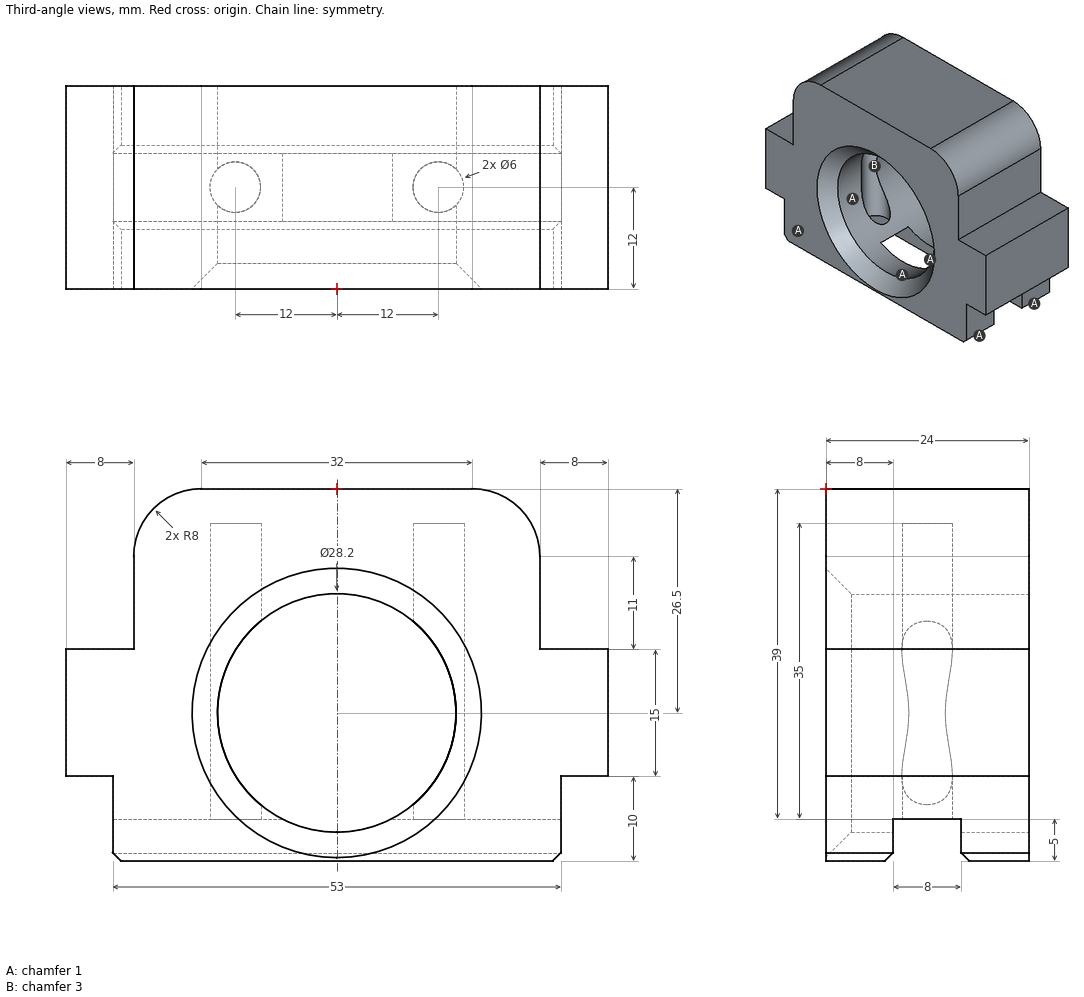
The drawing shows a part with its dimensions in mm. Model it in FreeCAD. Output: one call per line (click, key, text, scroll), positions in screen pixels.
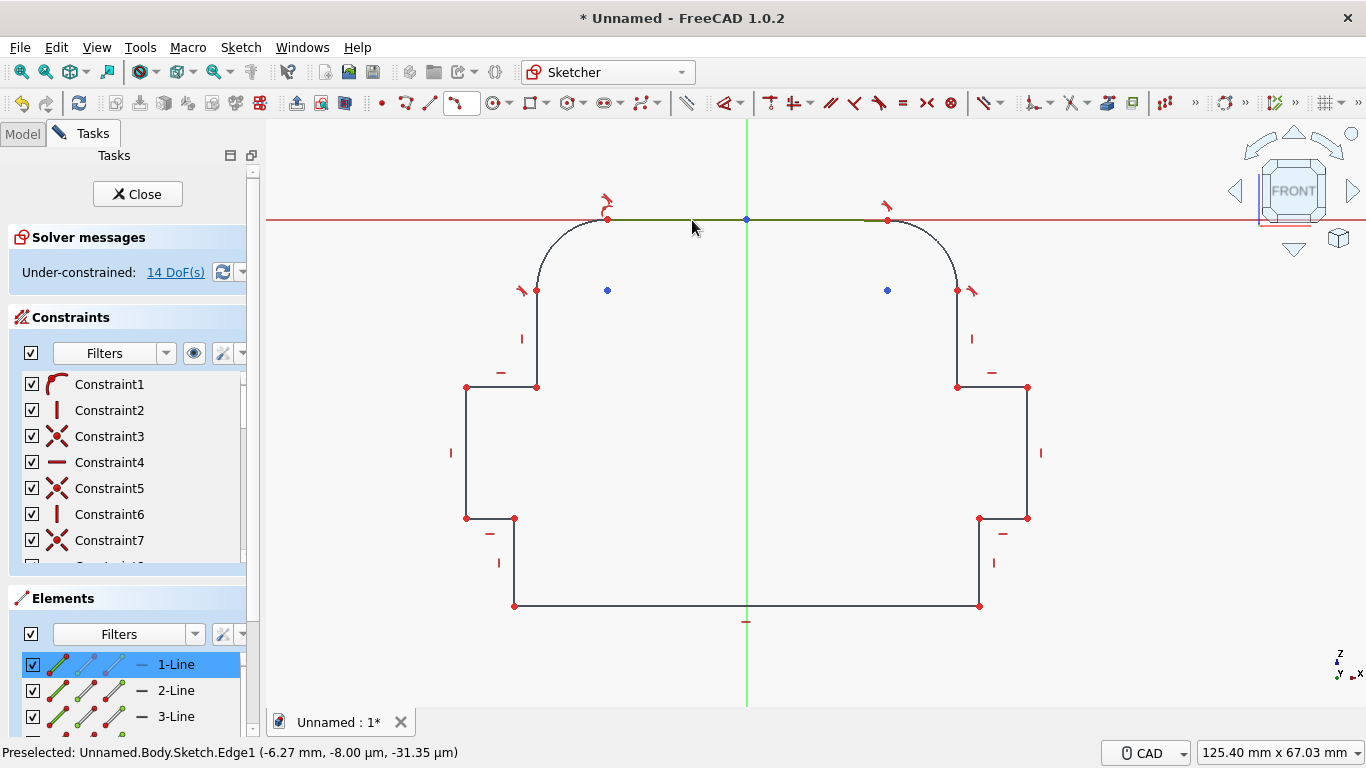
key(h)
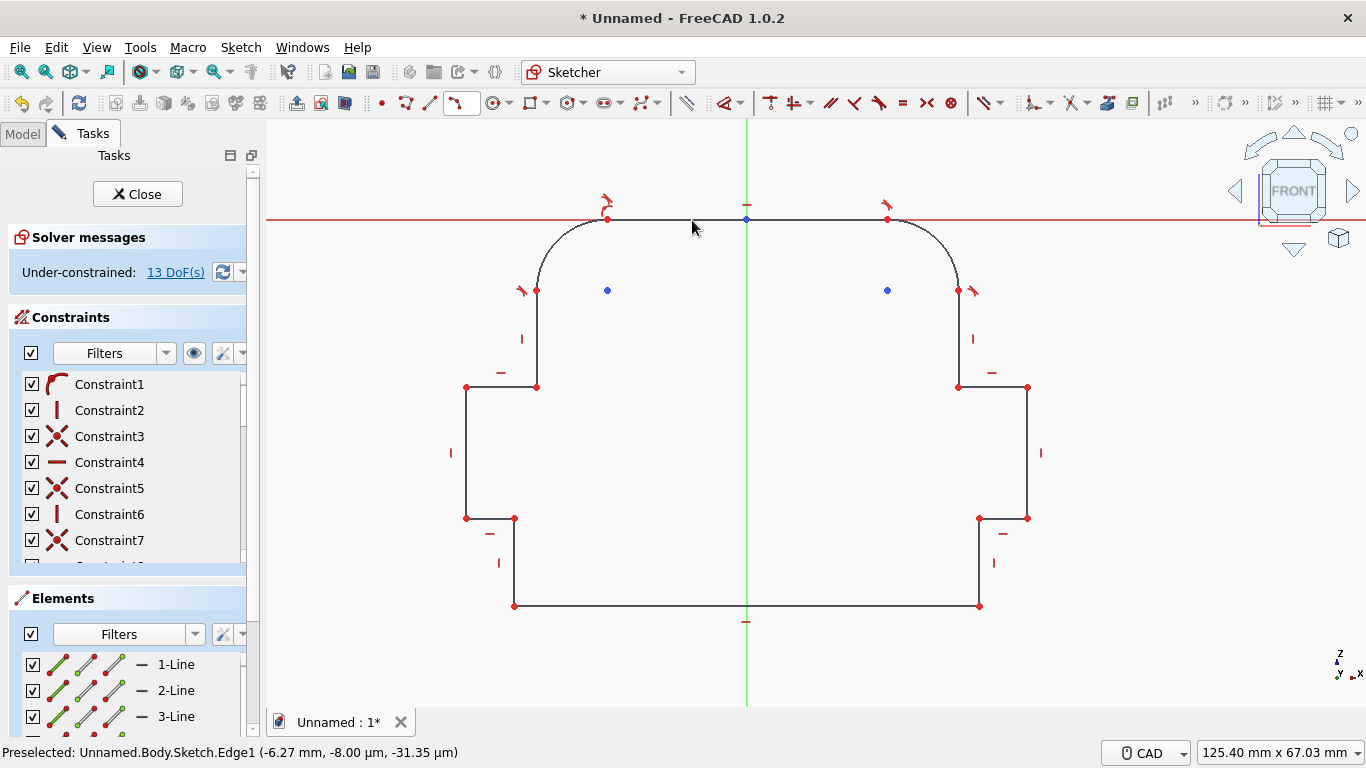
click(951, 258)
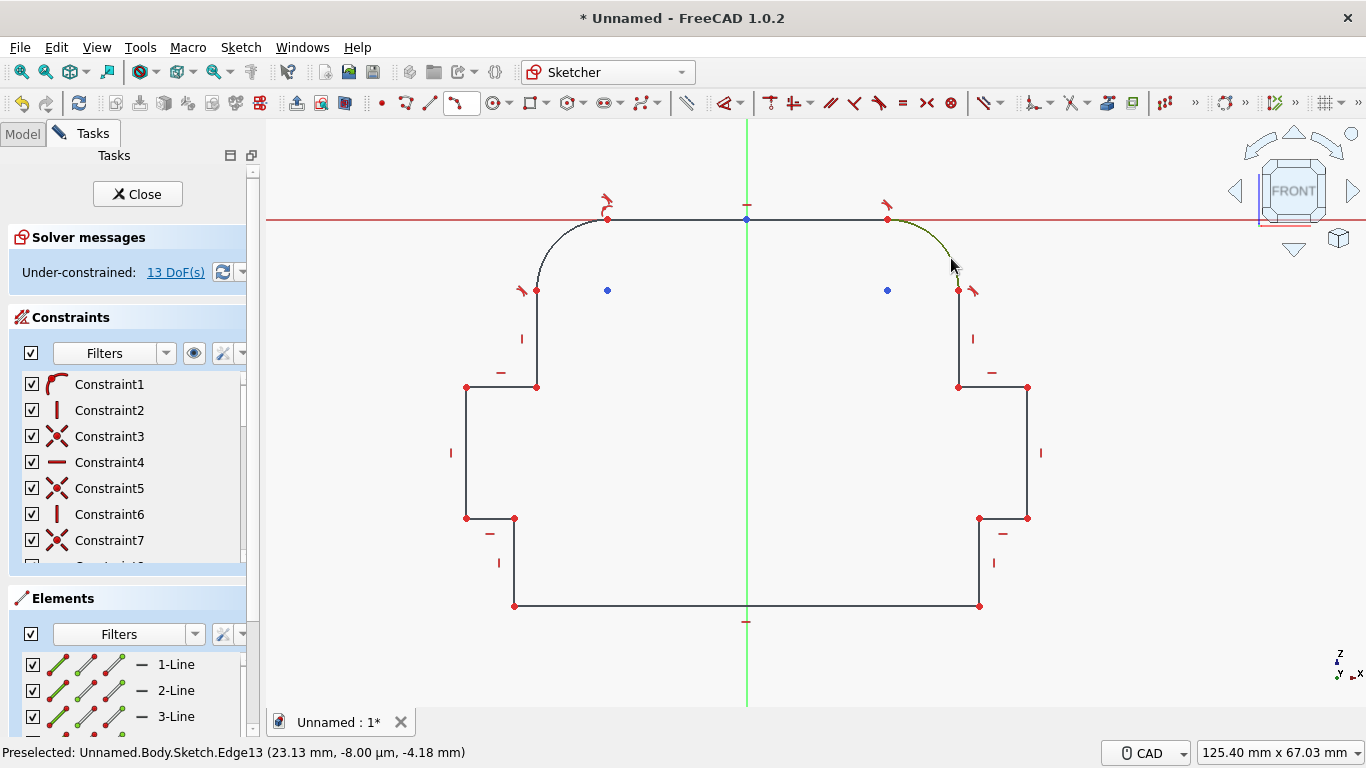
click(545, 258)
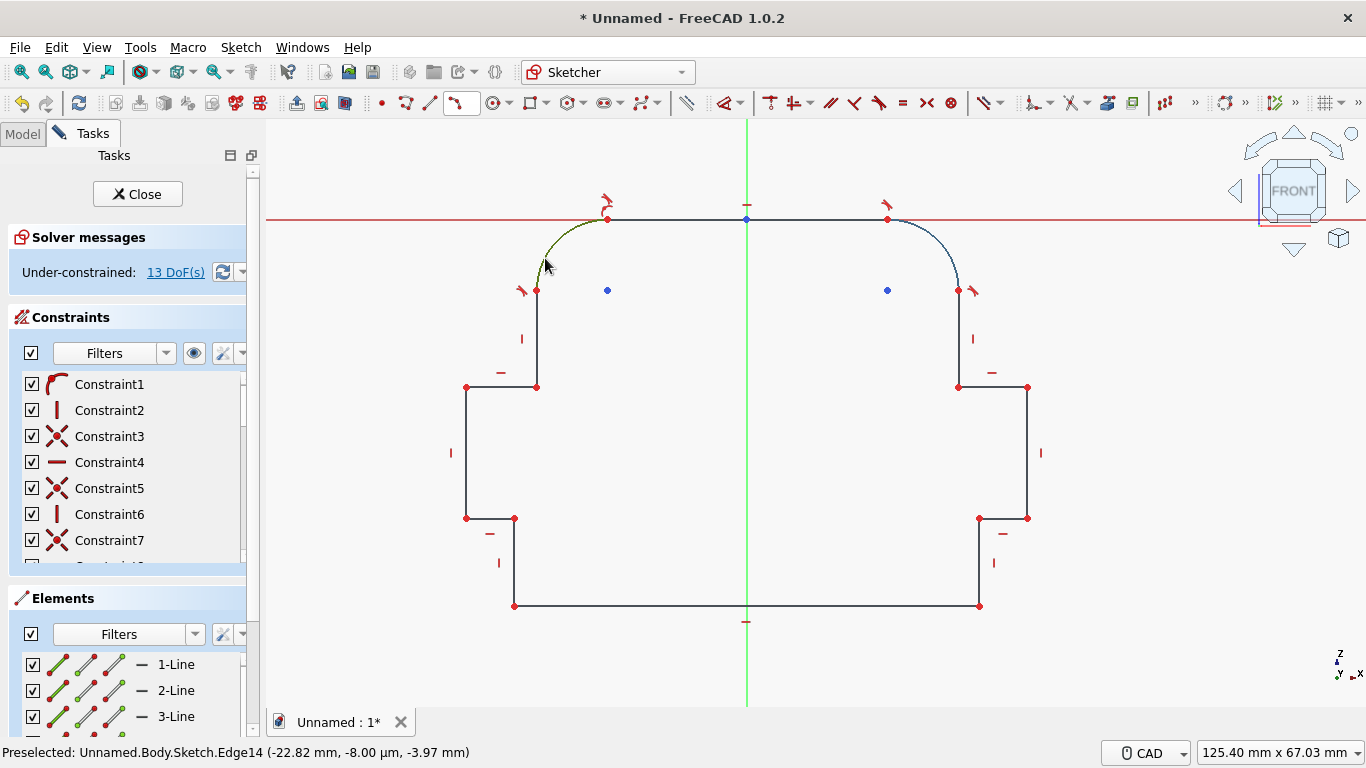
click(904, 104)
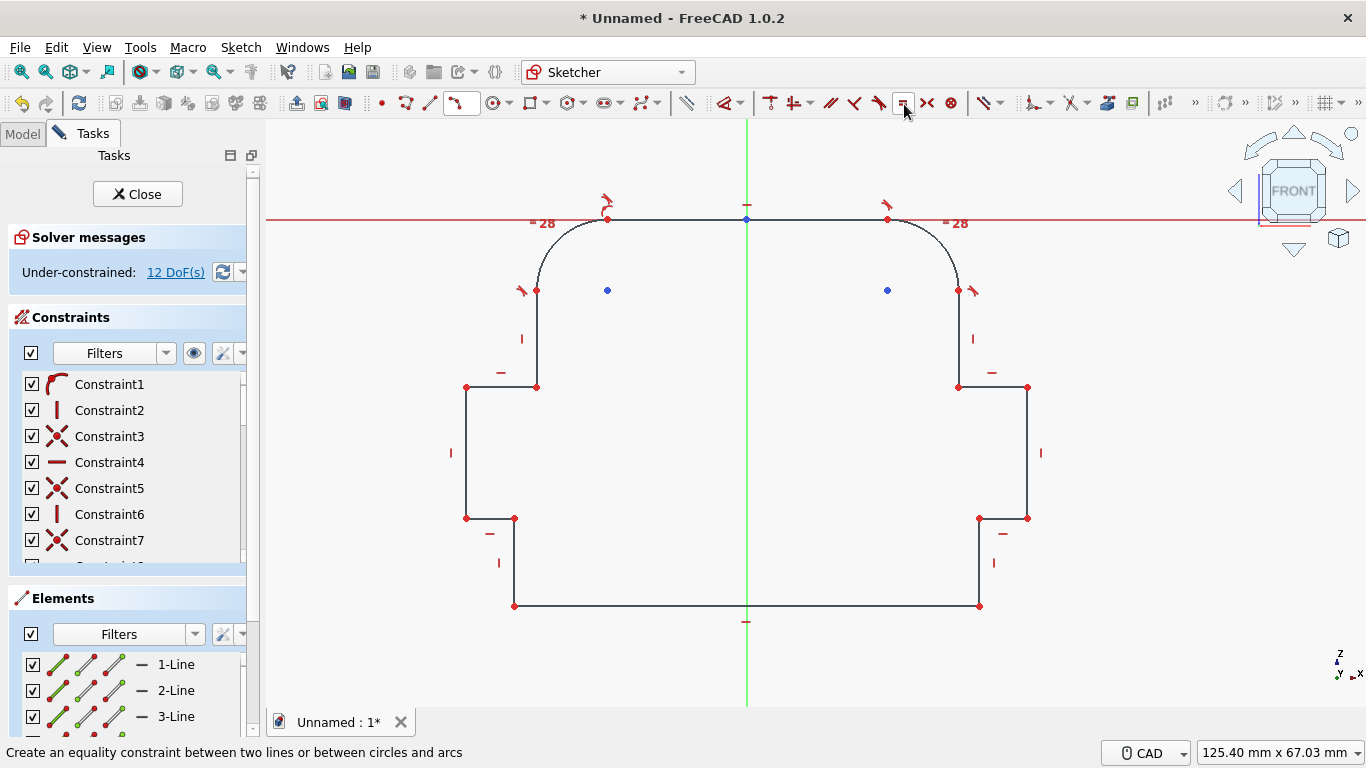
click(979, 519)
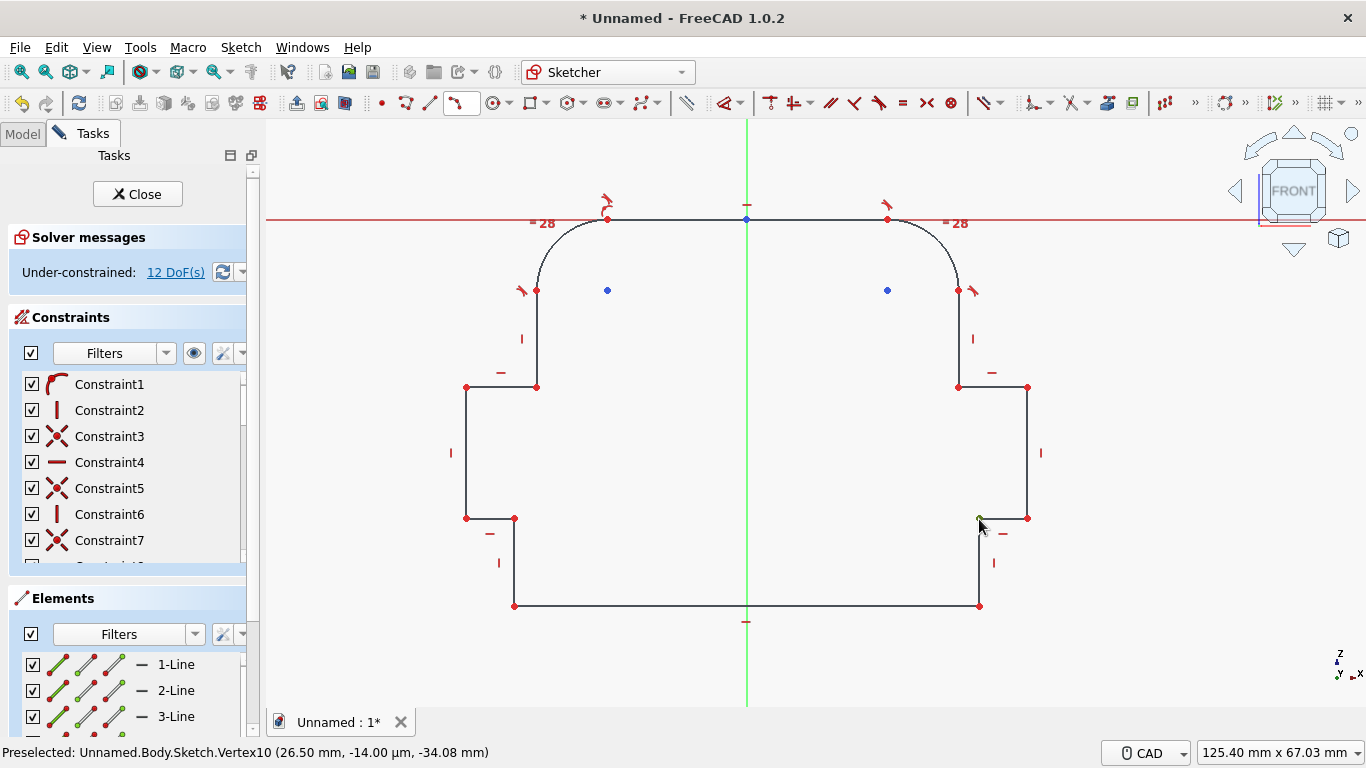
click(514, 519)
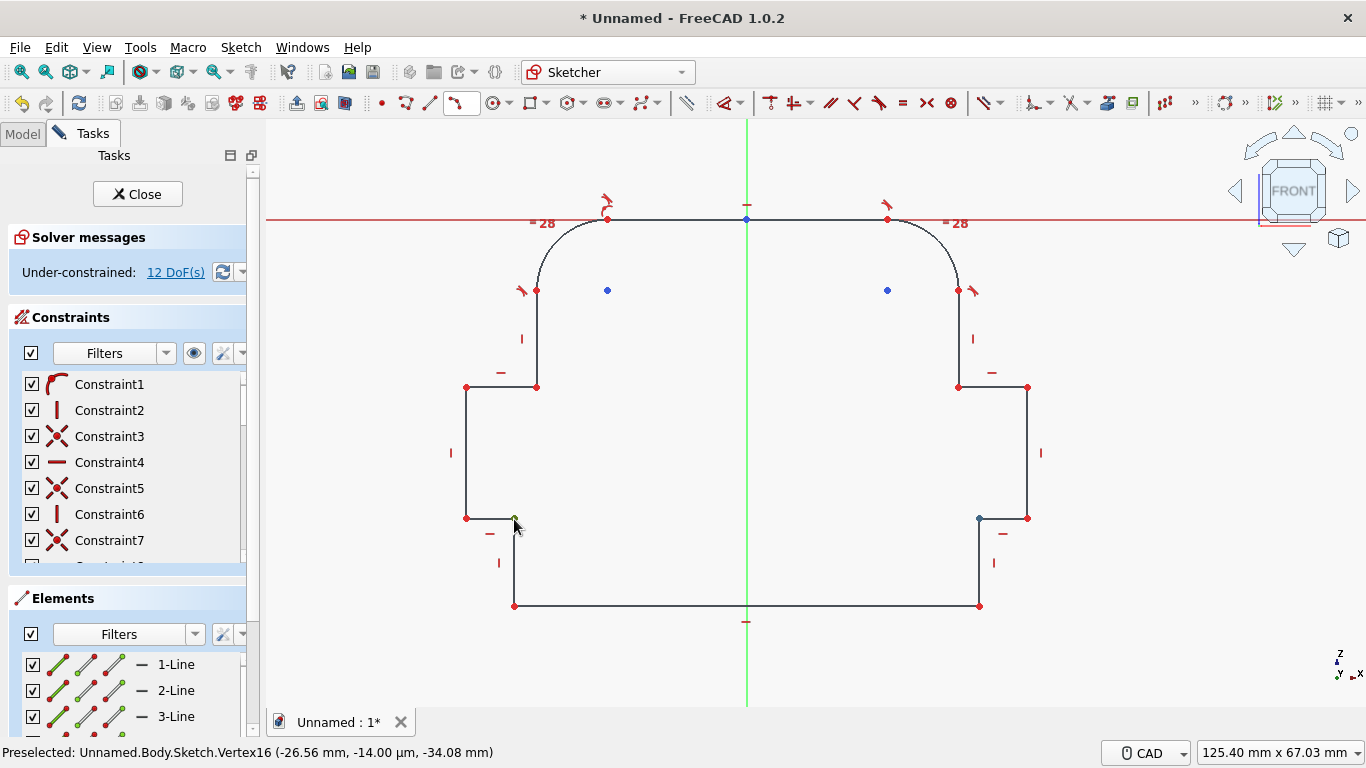
click(747, 641)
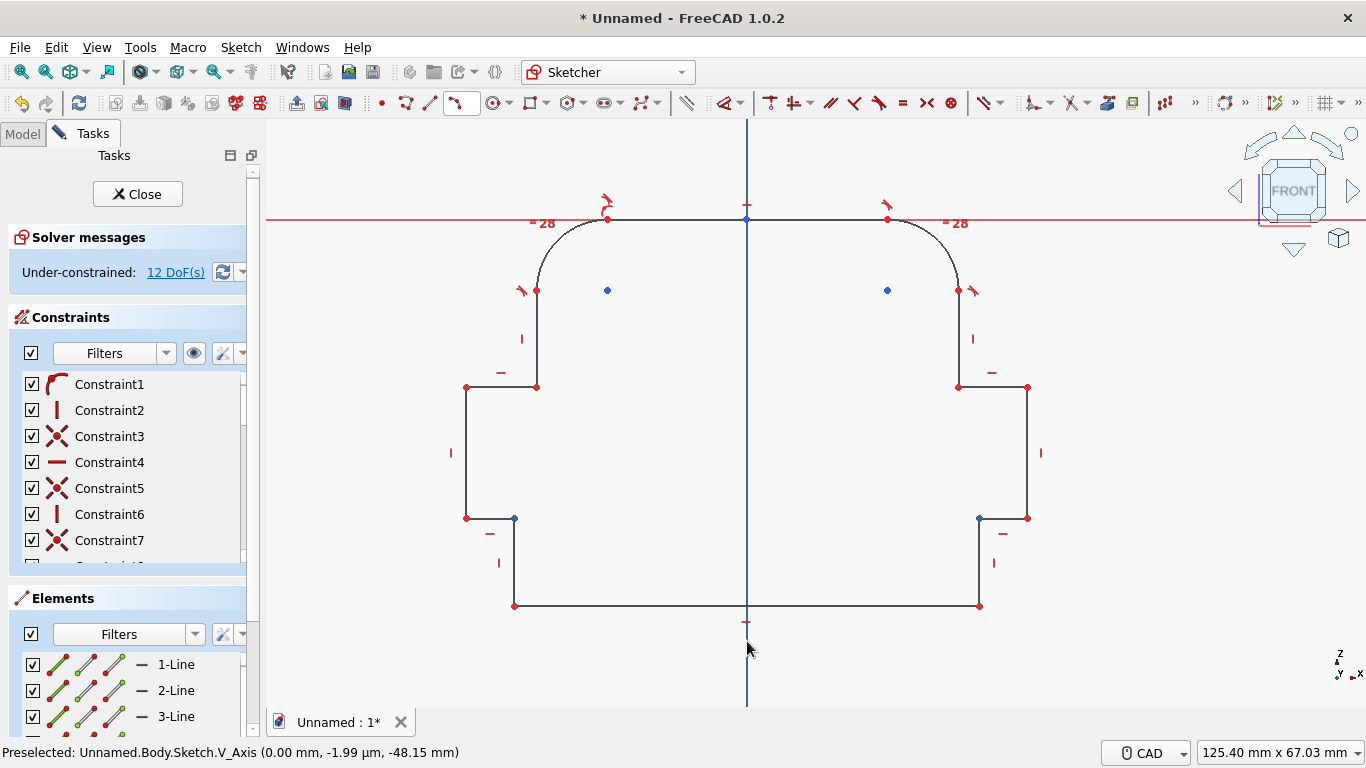
click(928, 104)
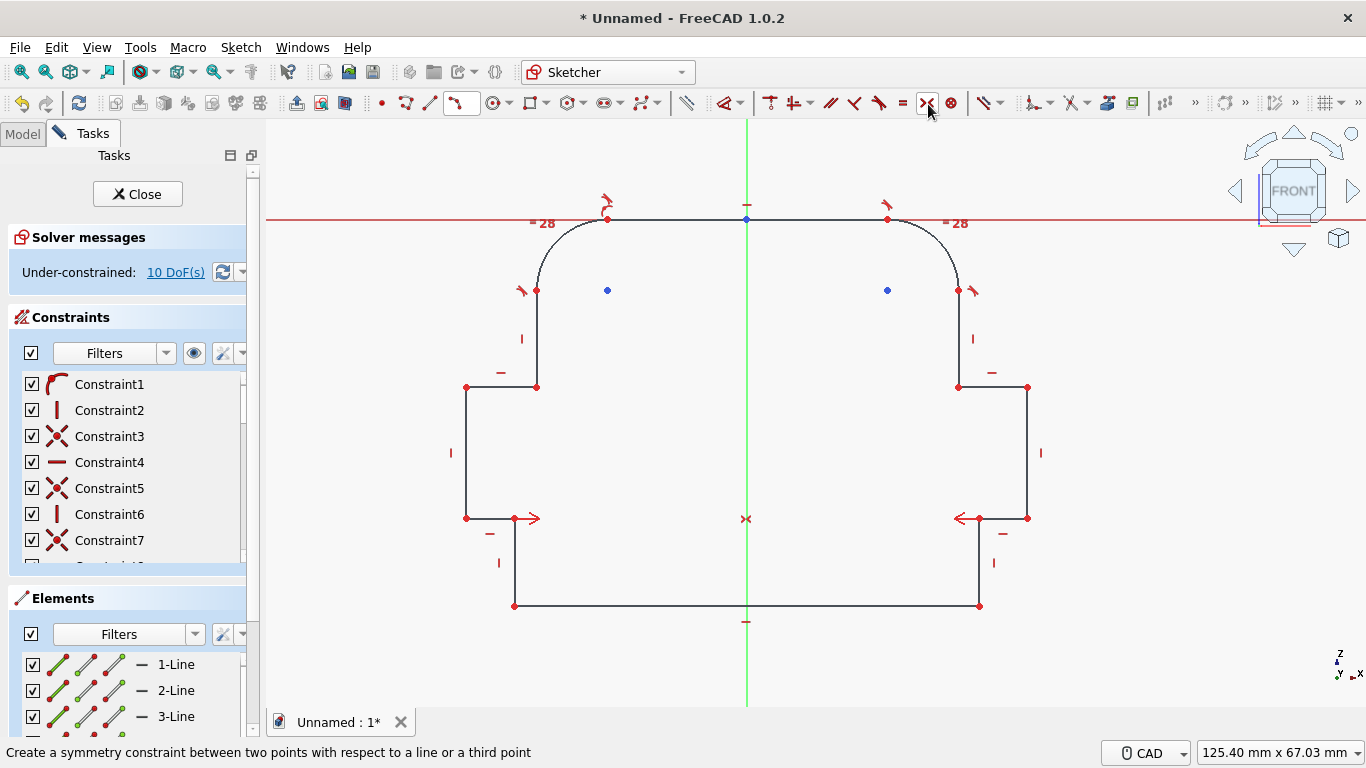
click(1027, 387)